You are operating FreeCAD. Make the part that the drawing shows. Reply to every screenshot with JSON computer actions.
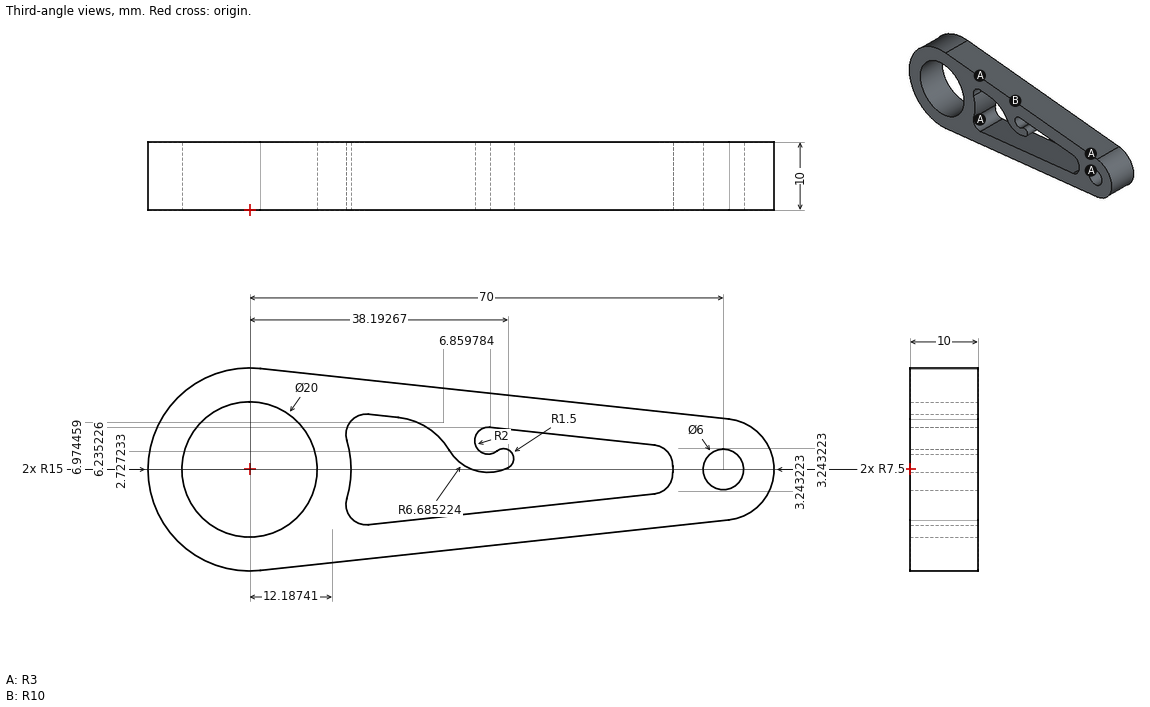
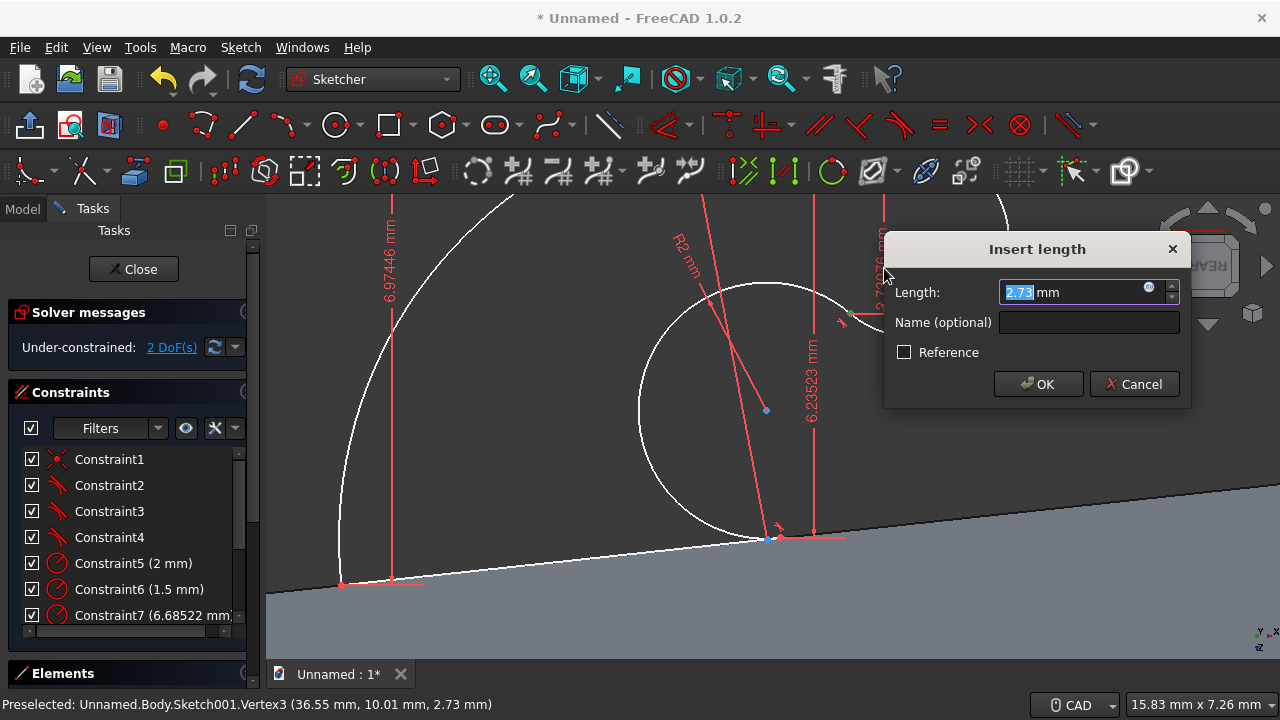
{"action": "type", "text": "2.727233"}
{"action": "key", "text": "Return"}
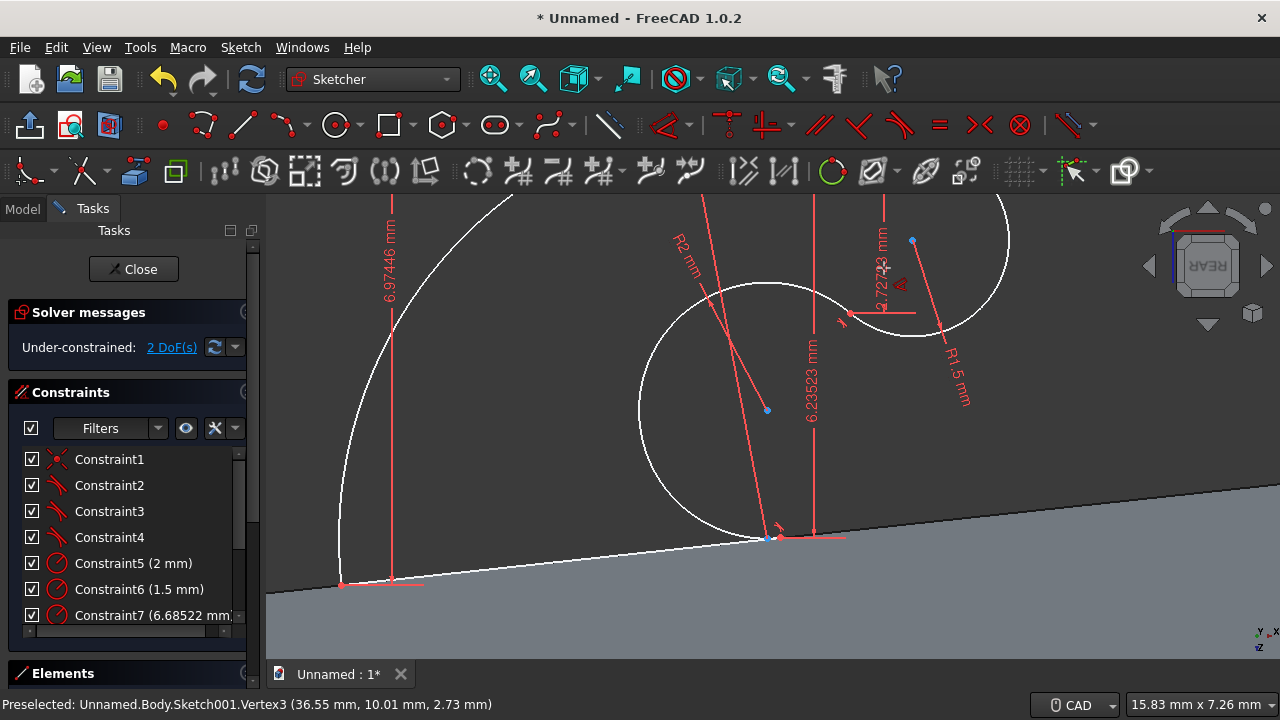
{"action": "scroll", "coordinate": [780, 542], "scroll_direction": "down", "scroll_amount": 2}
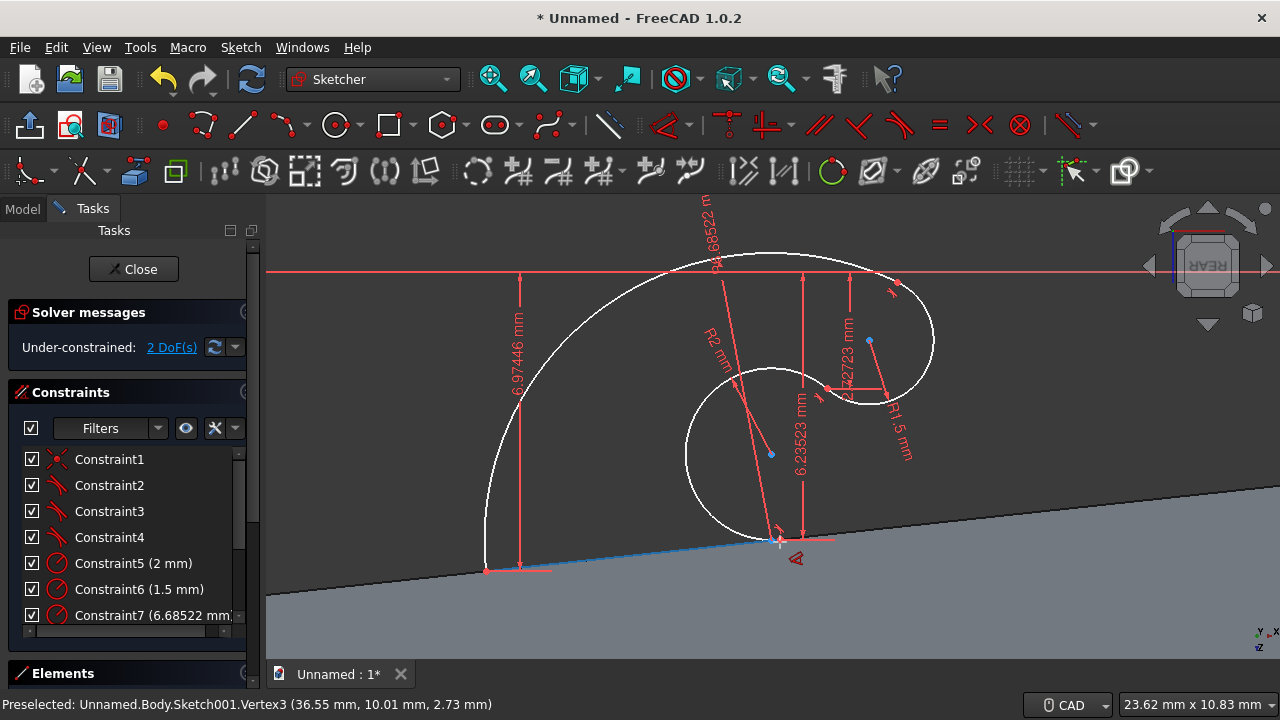
{"action": "left_click", "coordinate": [898, 282]}
{"action": "left_click", "coordinate": [596, 238]}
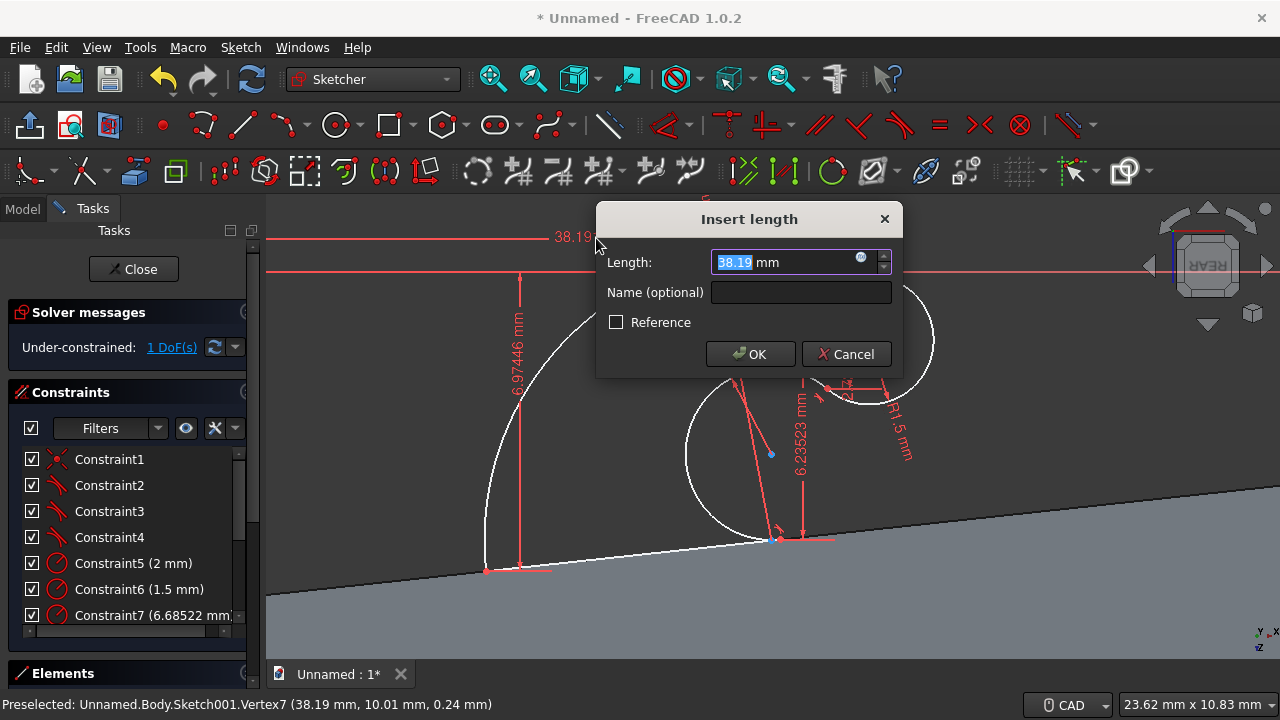
{"action": "type", "text": "38.19267"}
{"action": "key", "text": "Return"}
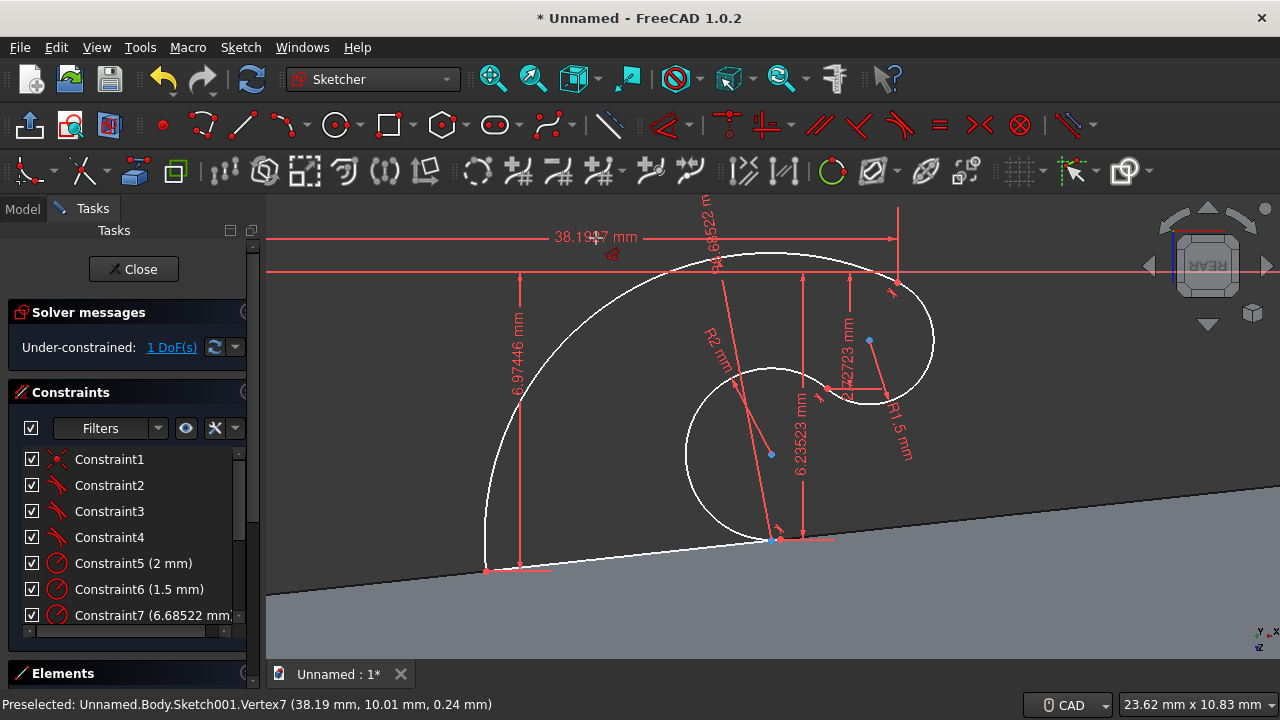
{"action": "left_click", "coordinate": [575, 562]}
{"action": "left_click", "coordinate": [634, 605]}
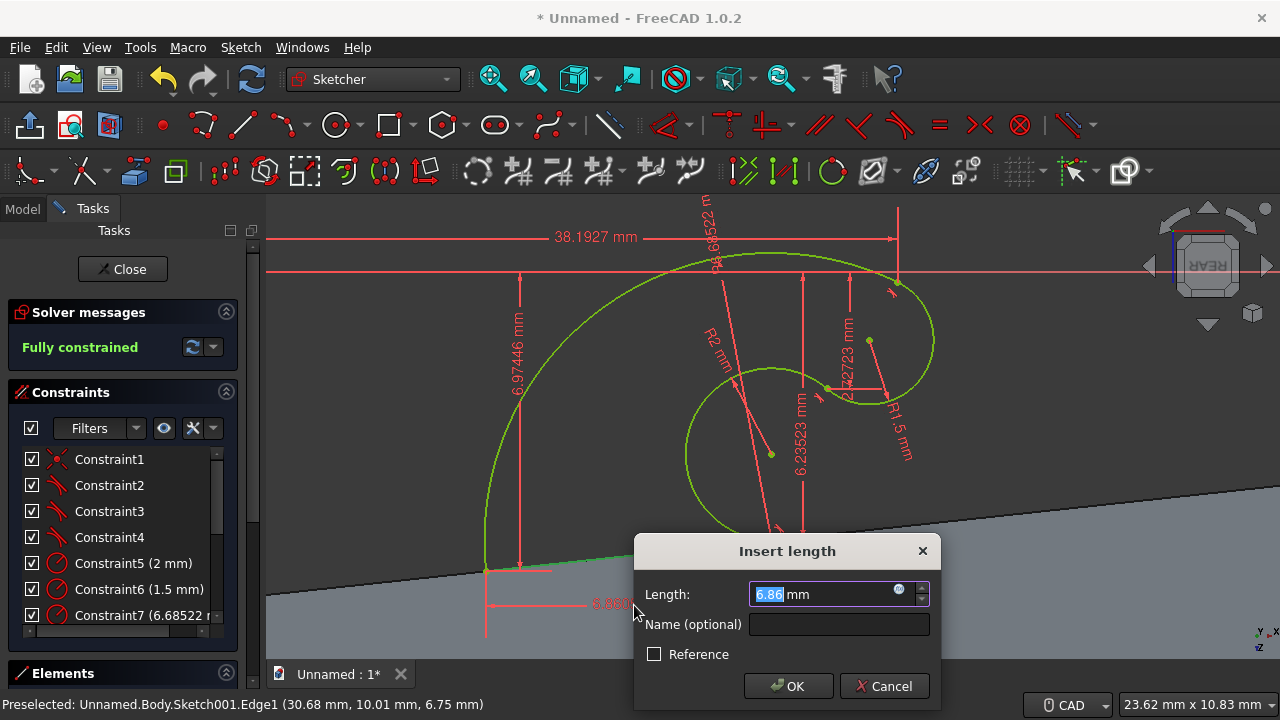
{"action": "type", "text": "6.859784"}
{"action": "key", "text": "Return"}
{"action": "key", "text": "Escape"}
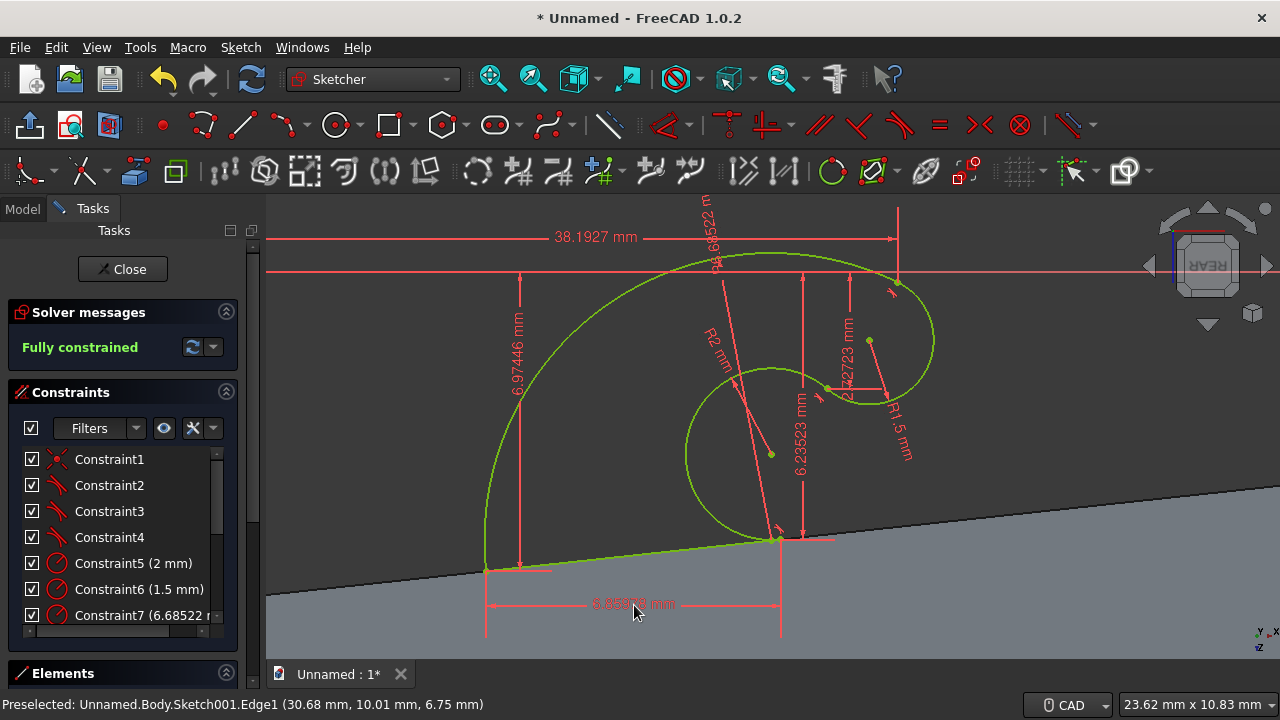
{"action": "left_click", "coordinate": [123, 269]}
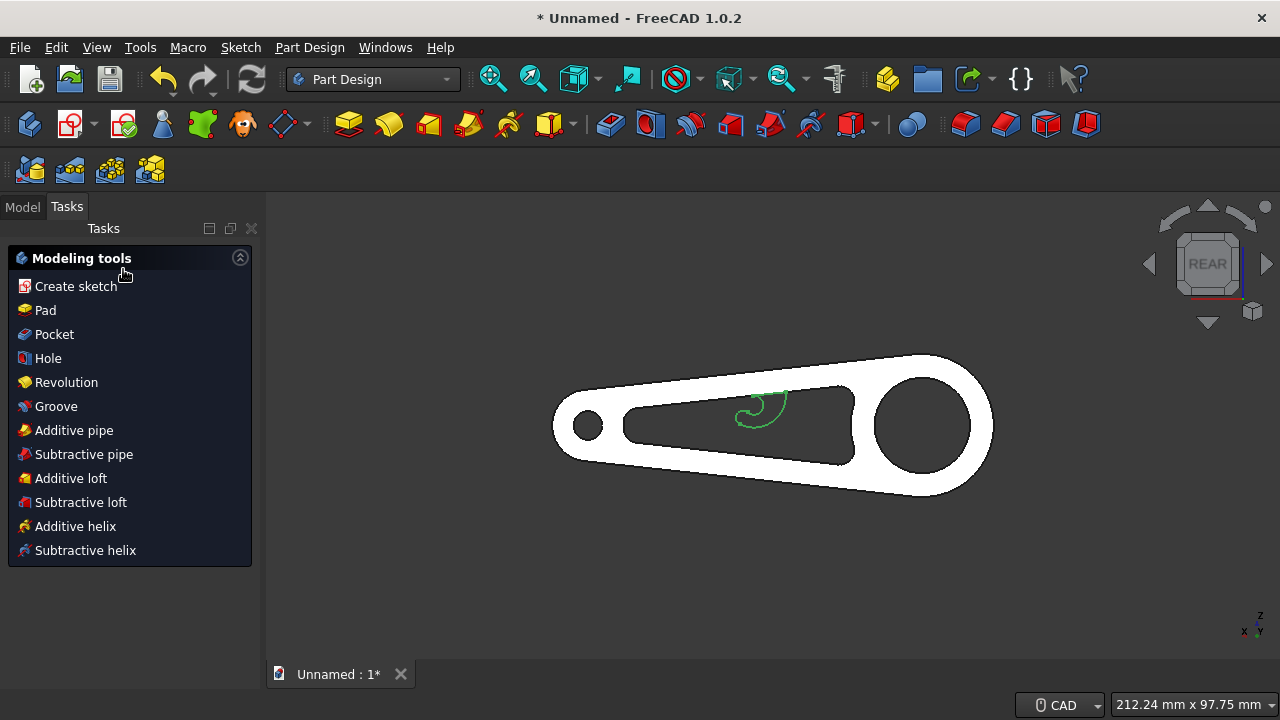
{"action": "left_click", "coordinate": [350, 124]}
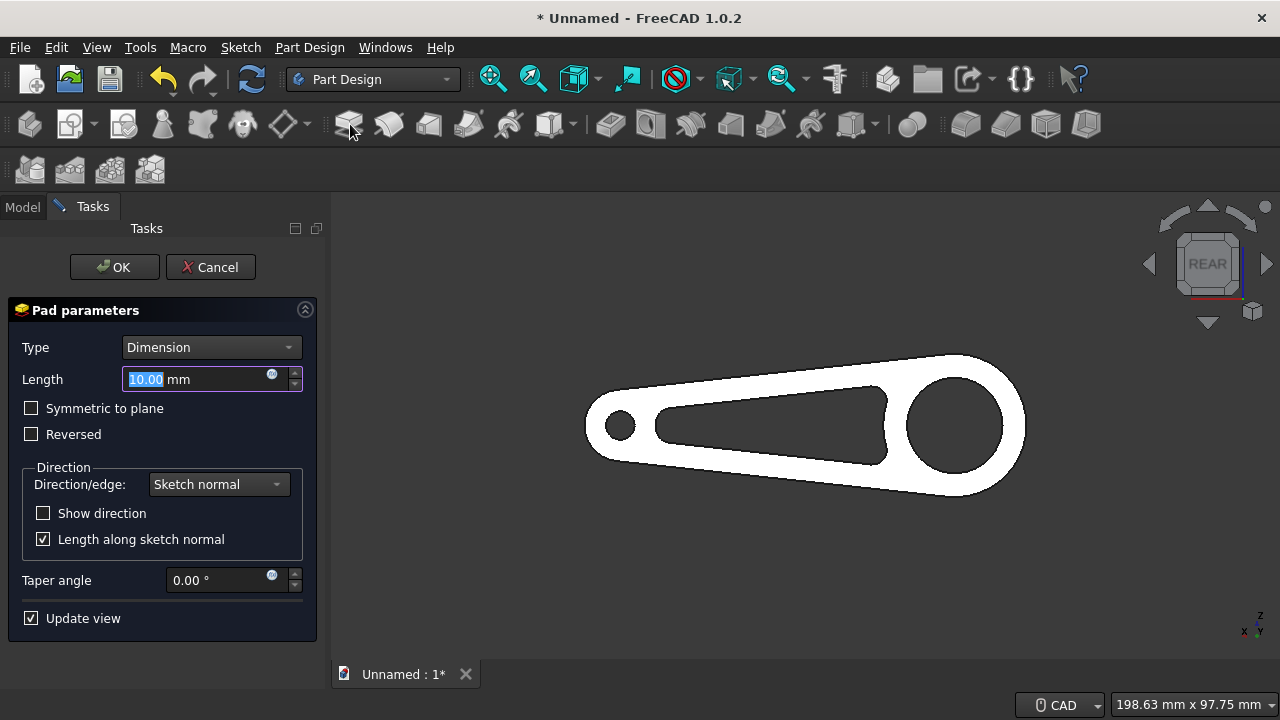
{"action": "type", "text": "10"}
{"action": "key", "text": "Tab"}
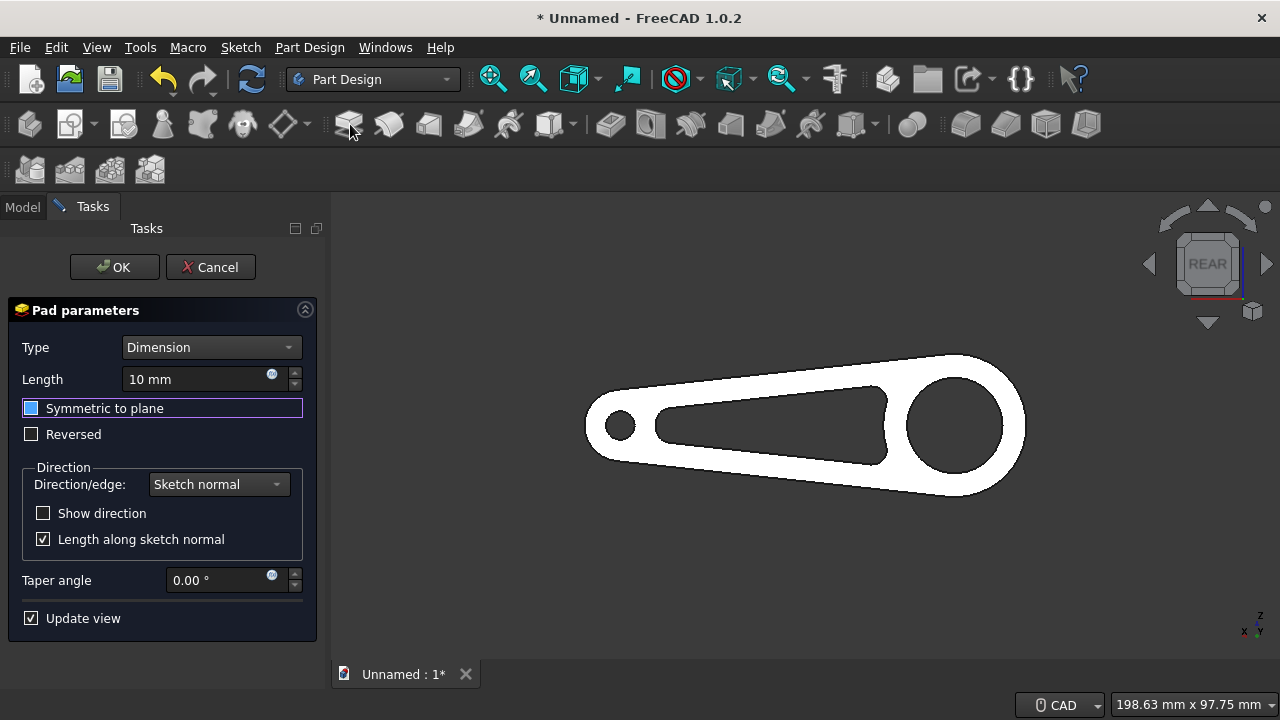
{"action": "left_click", "coordinate": [30, 434]}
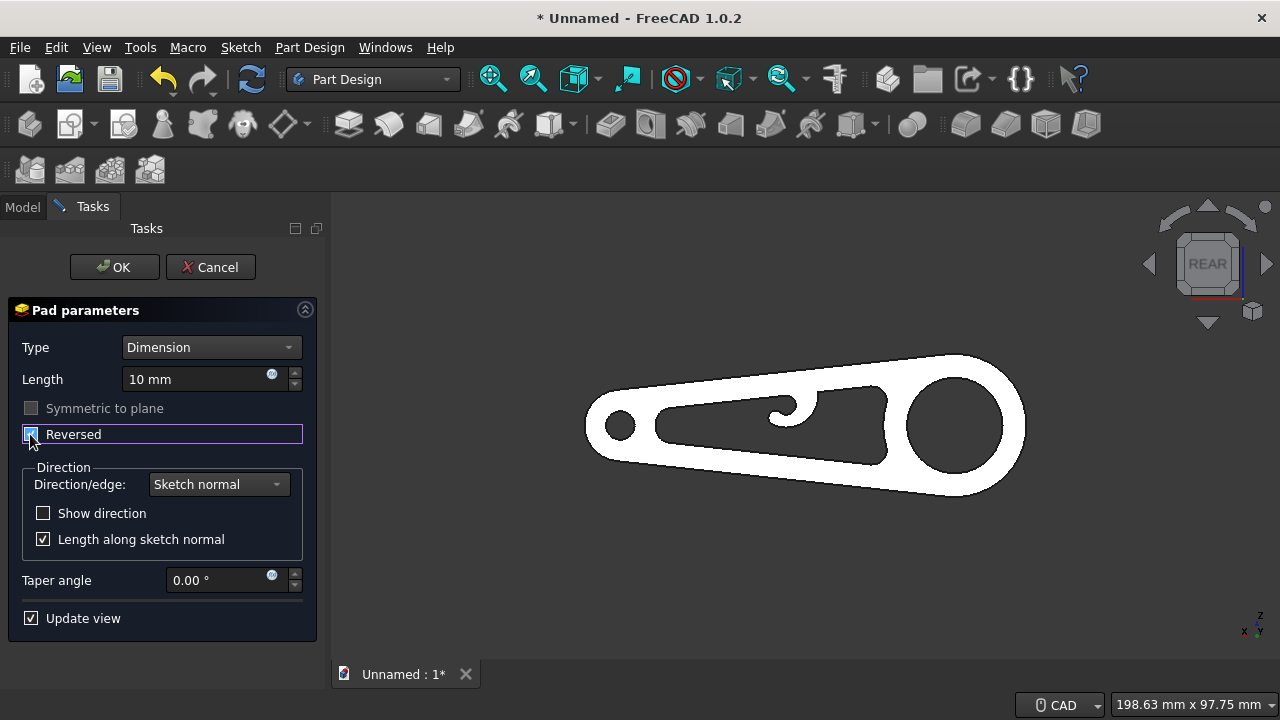
{"action": "left_click", "coordinate": [115, 267]}